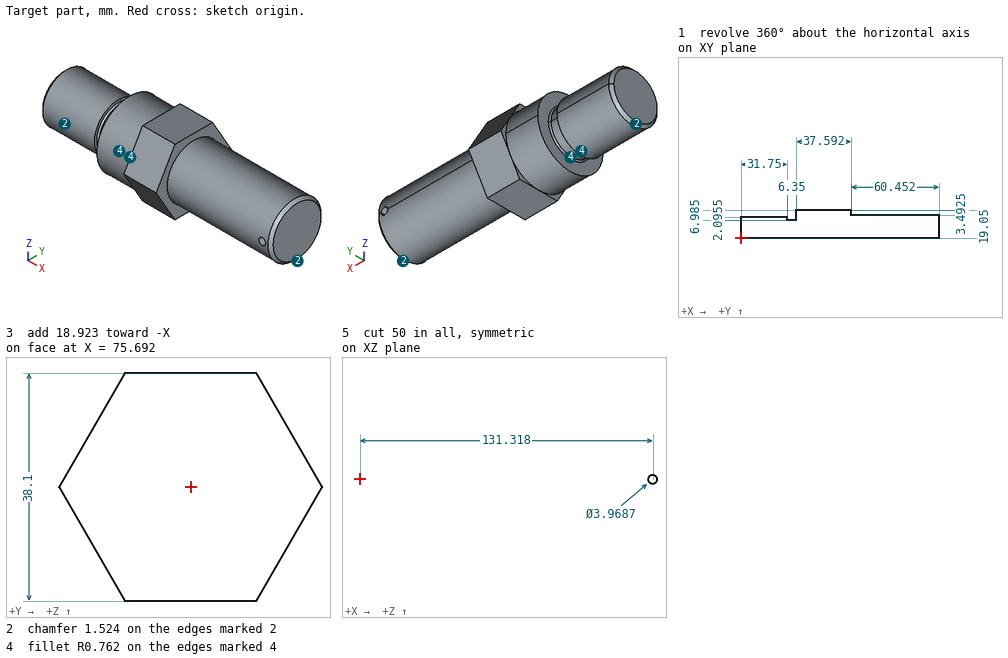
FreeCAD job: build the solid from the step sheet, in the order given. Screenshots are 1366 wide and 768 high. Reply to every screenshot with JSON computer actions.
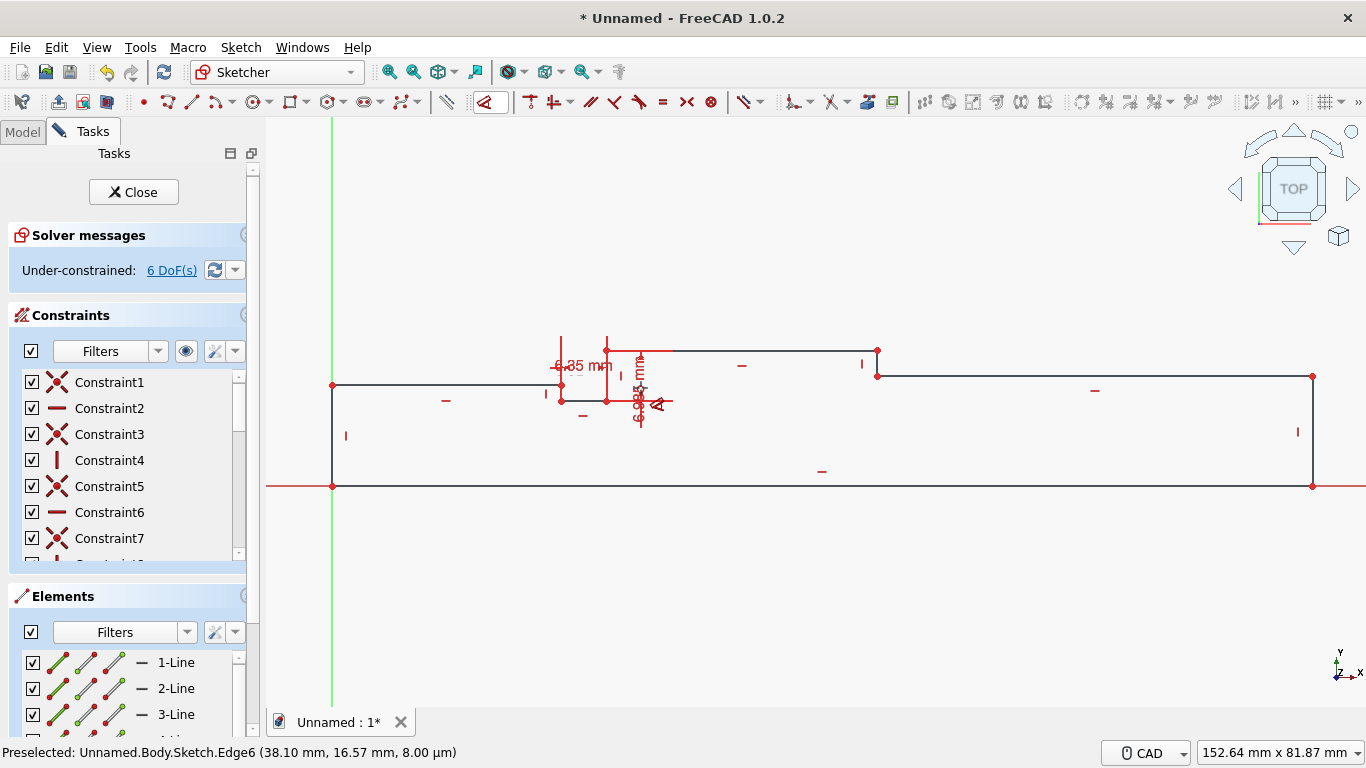
{"action": "left_click", "coordinate": [492, 385]}
{"action": "left_click", "coordinate": [447, 351]}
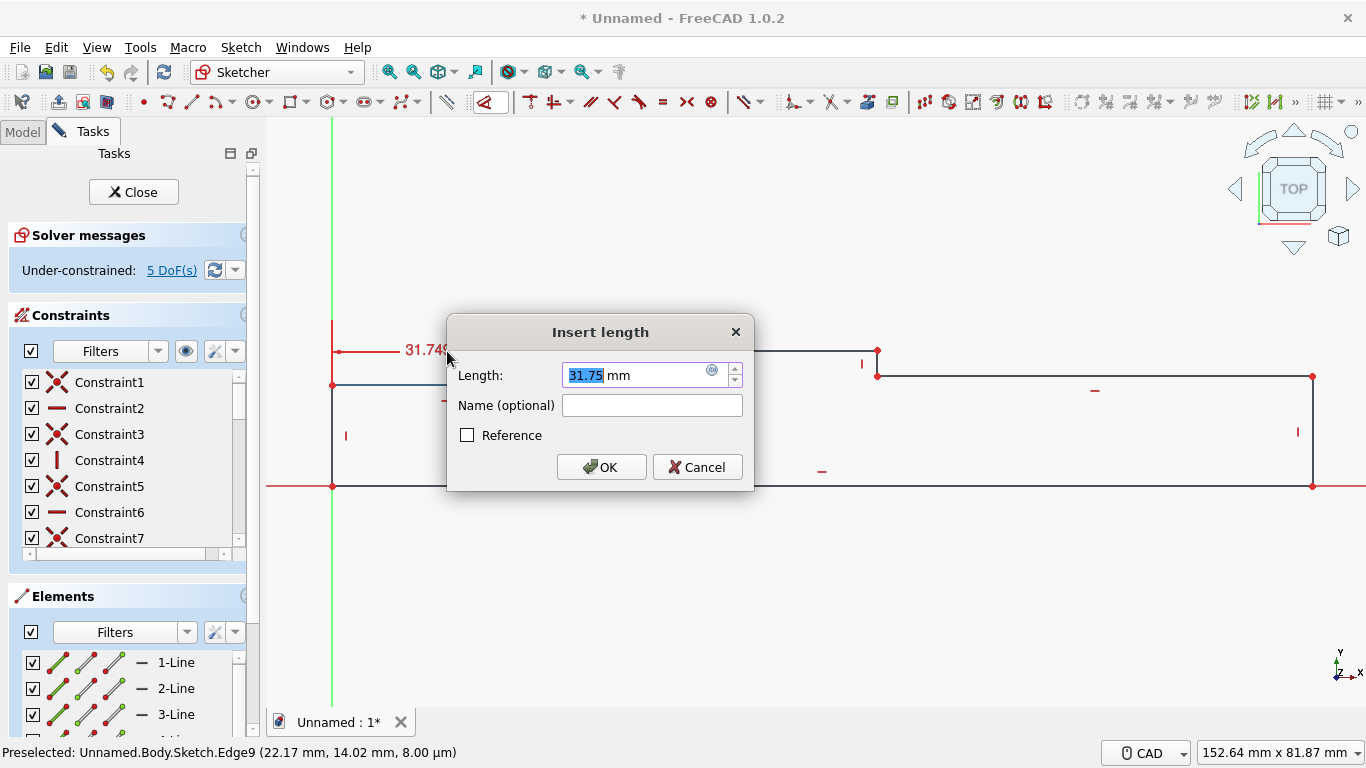
{"action": "type", "text": "31.75"}
{"action": "key", "text": "Return"}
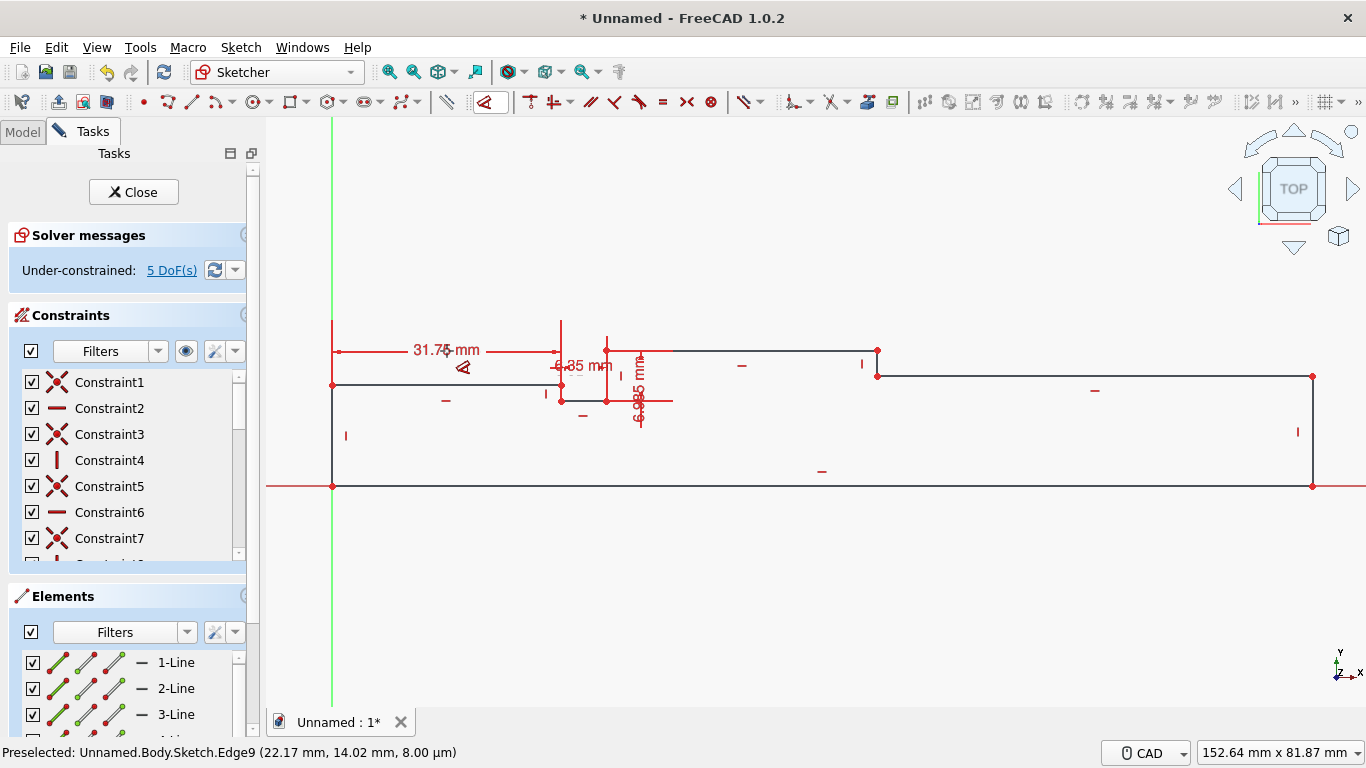
{"action": "left_click", "coordinate": [1182, 376]}
{"action": "left_click", "coordinate": [1039, 342]}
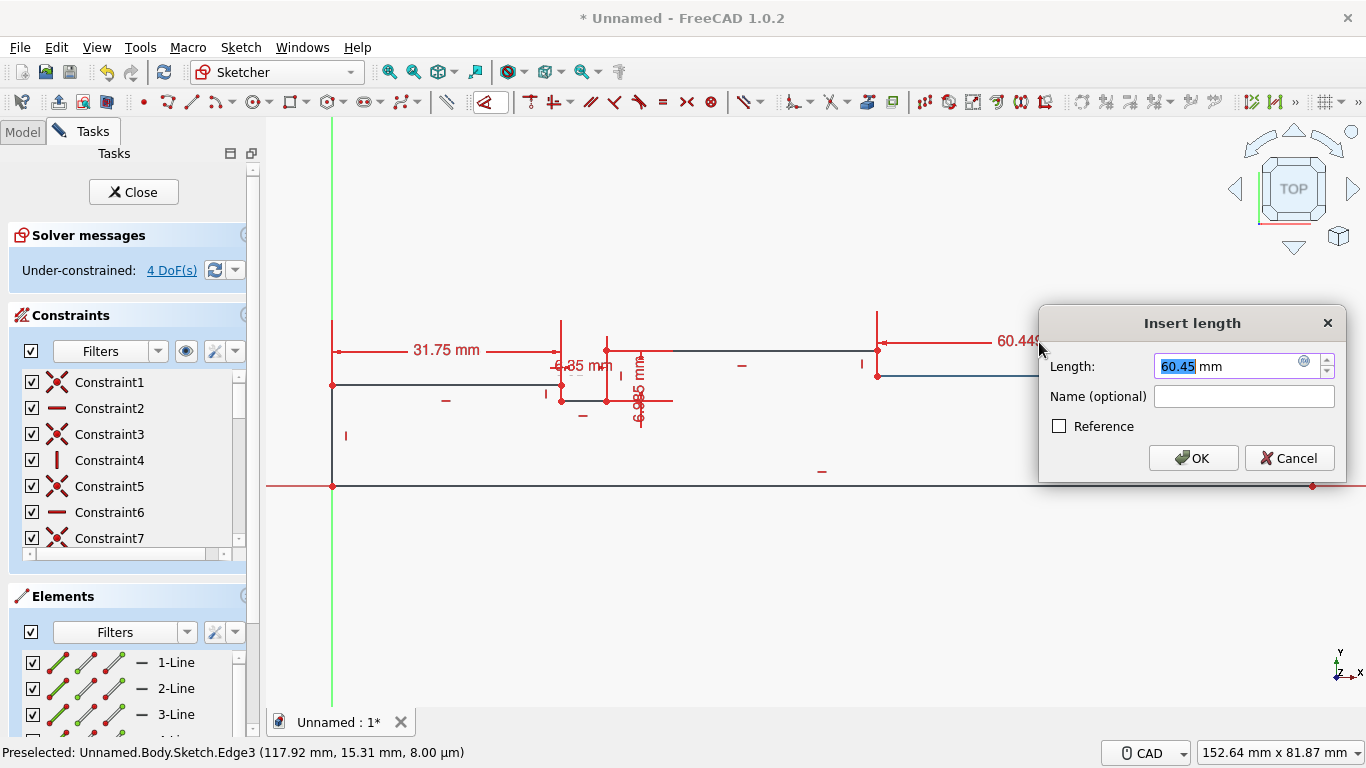
{"action": "type", "text": "60.452"}
{"action": "key", "text": "Return"}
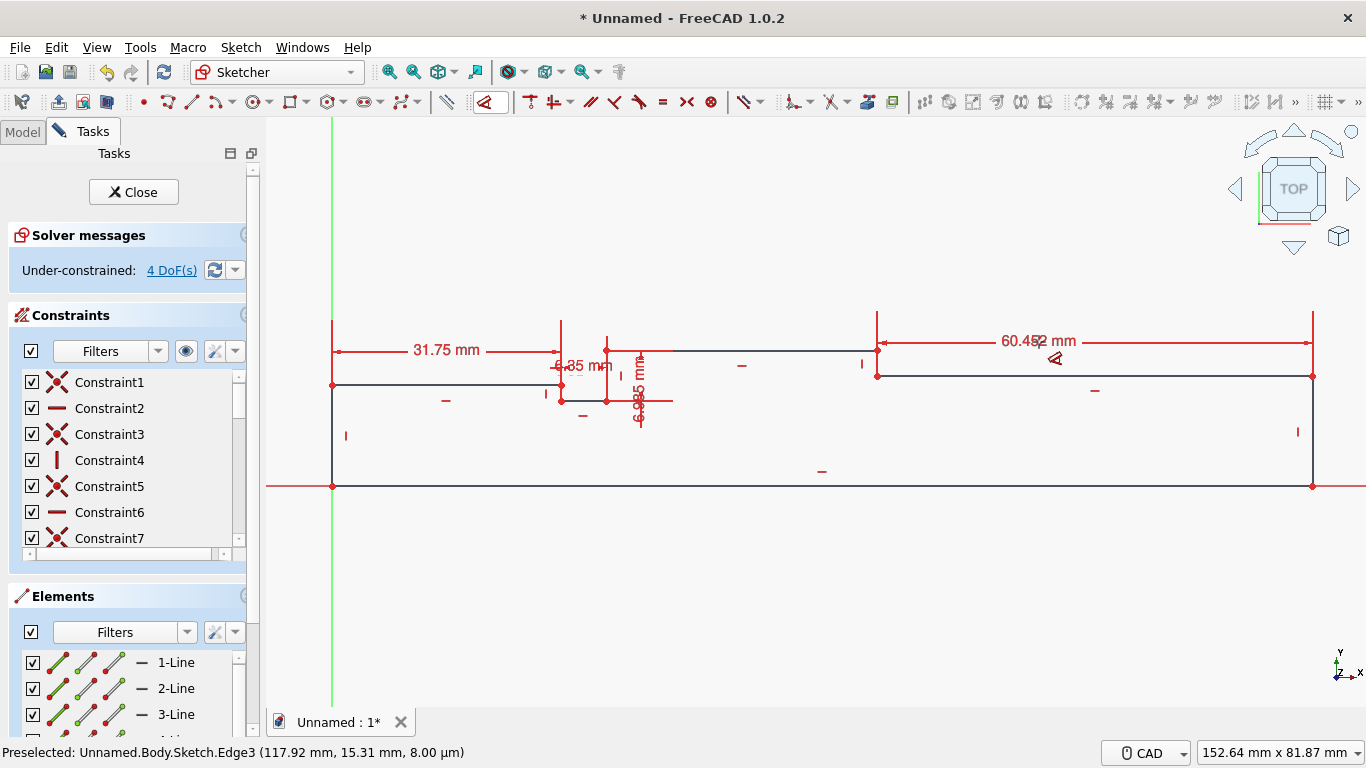
{"action": "scroll", "coordinate": [877, 366], "scroll_direction": "up", "scroll_amount": 3}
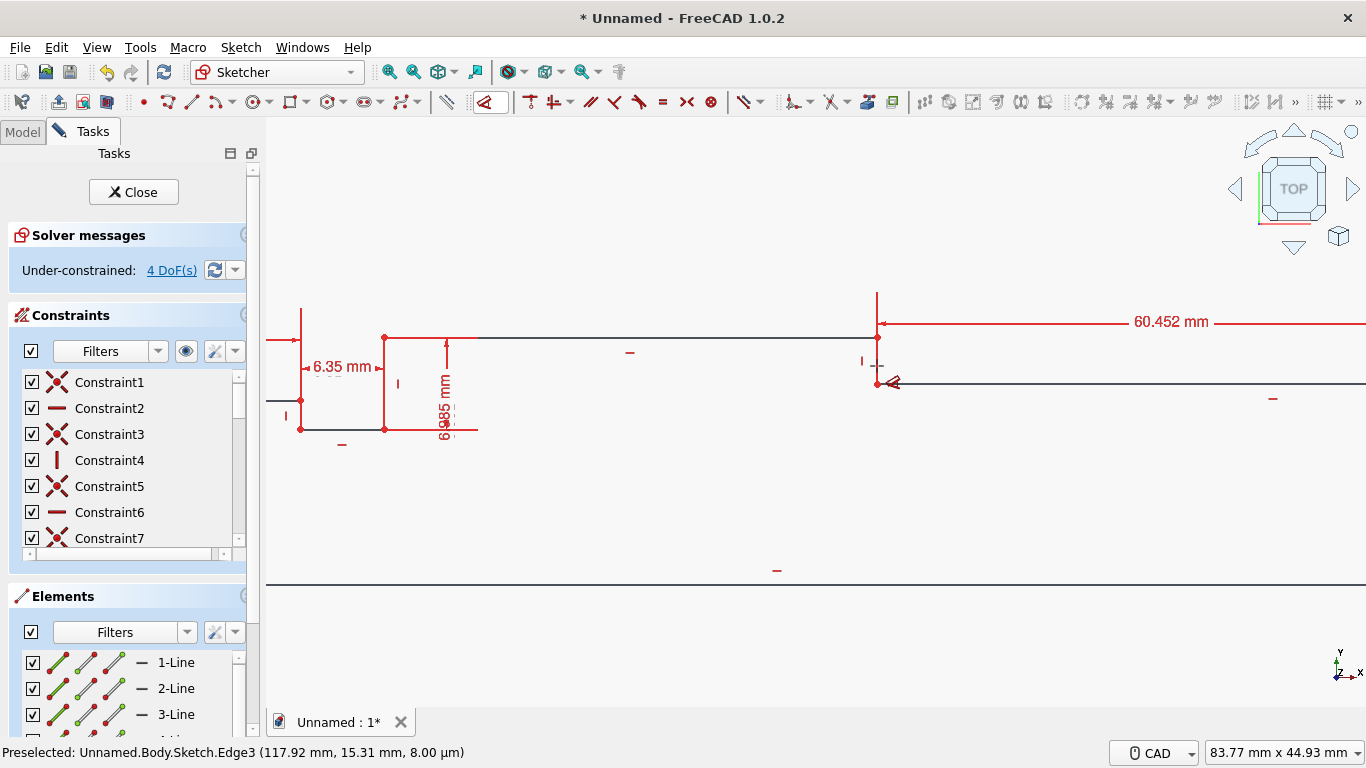
{"action": "left_click", "coordinate": [877, 366]}
{"action": "left_click", "coordinate": [911, 361]}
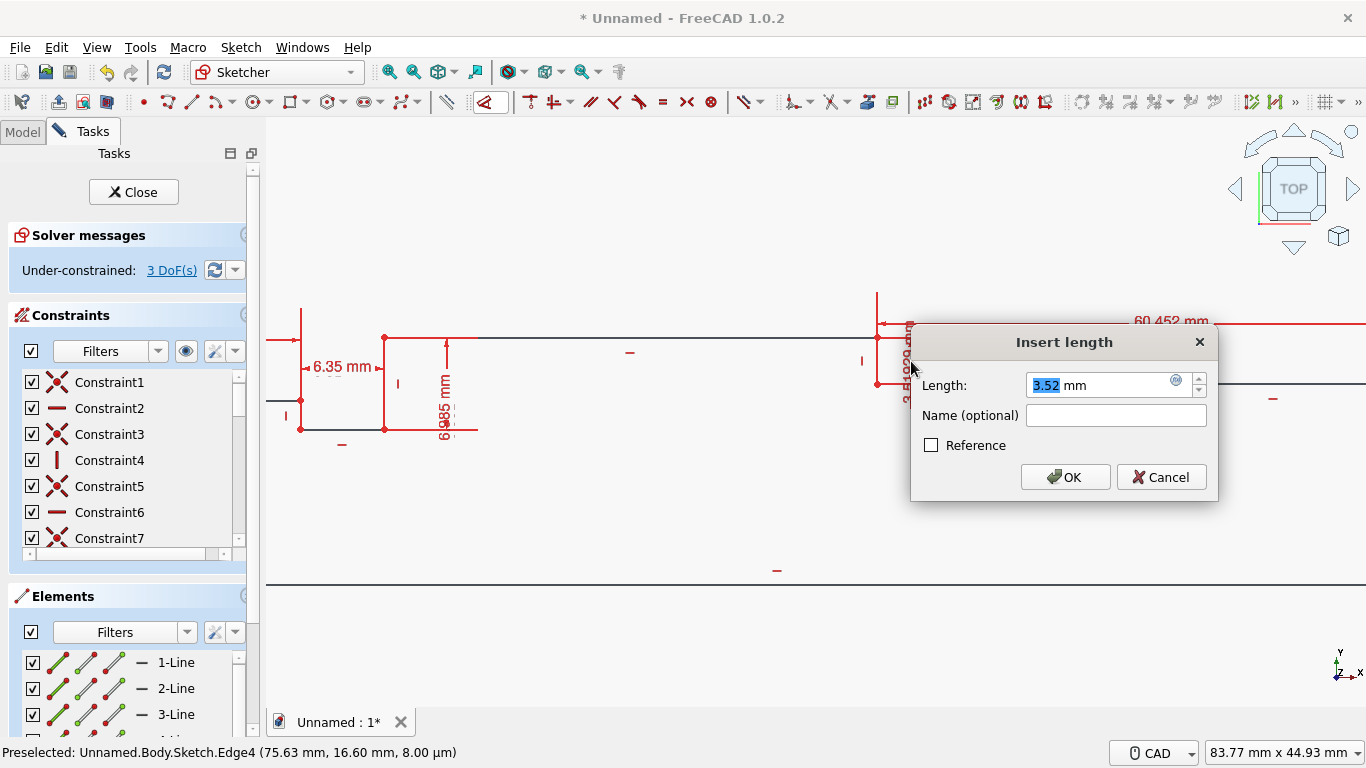
{"action": "type", "text": "3.4925"}
{"action": "key", "text": "Return"}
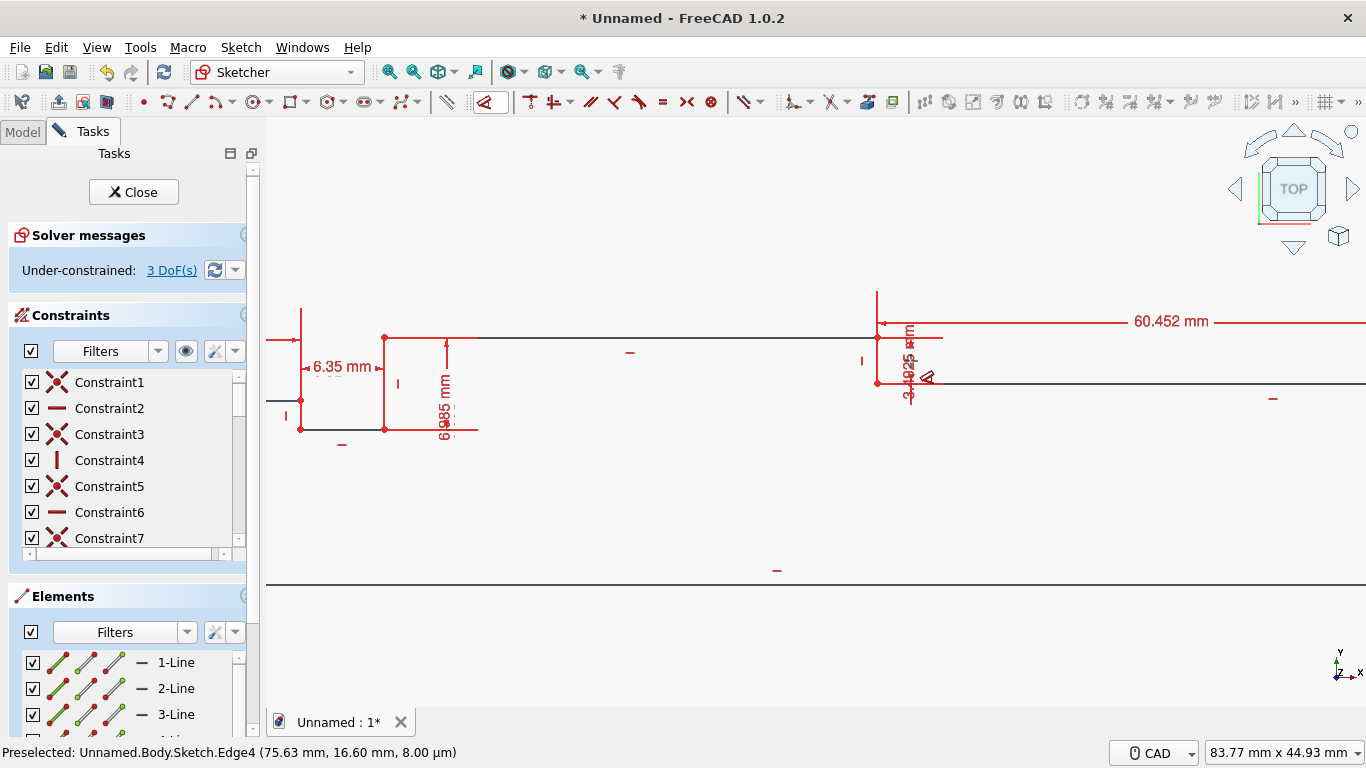
{"action": "left_click", "coordinate": [729, 338]}
{"action": "left_click", "coordinate": [631, 304]}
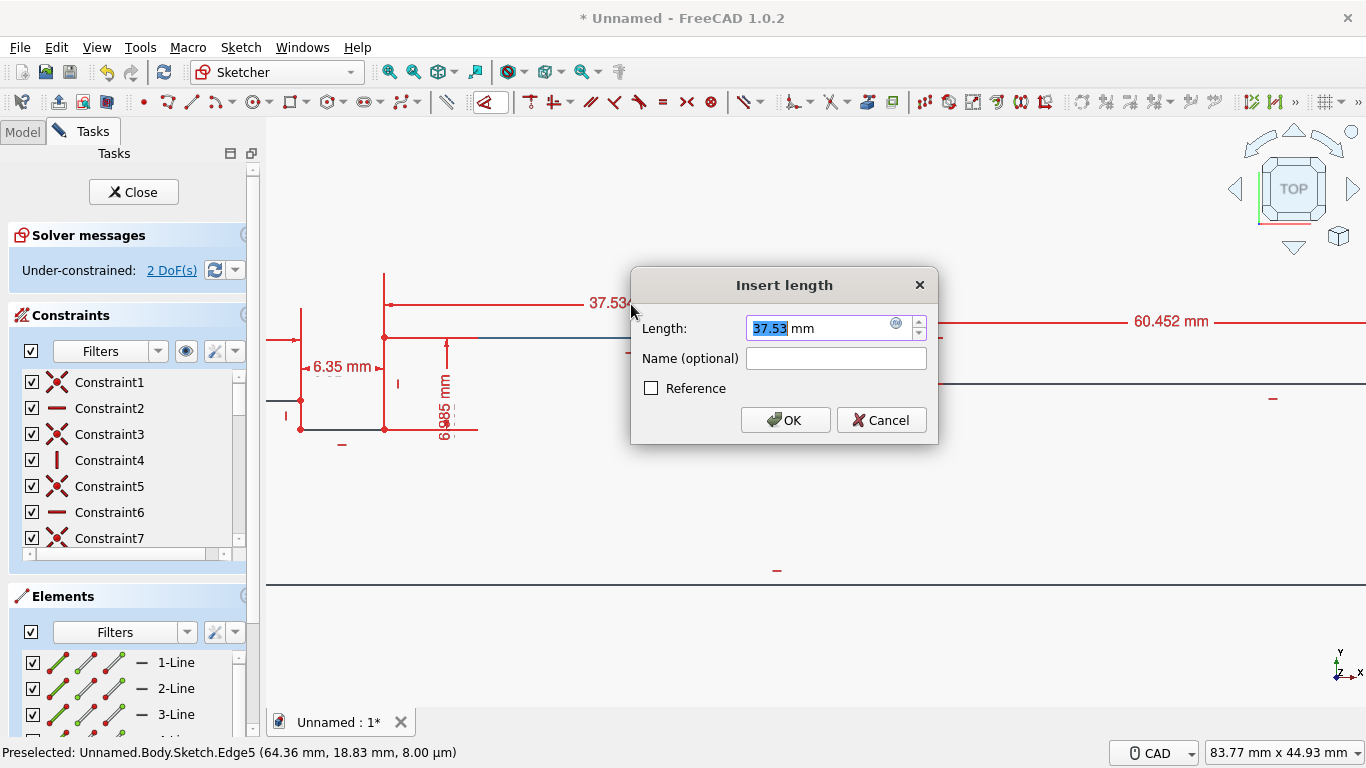
{"action": "type", "text": "37.592"}
{"action": "key", "text": "Return"}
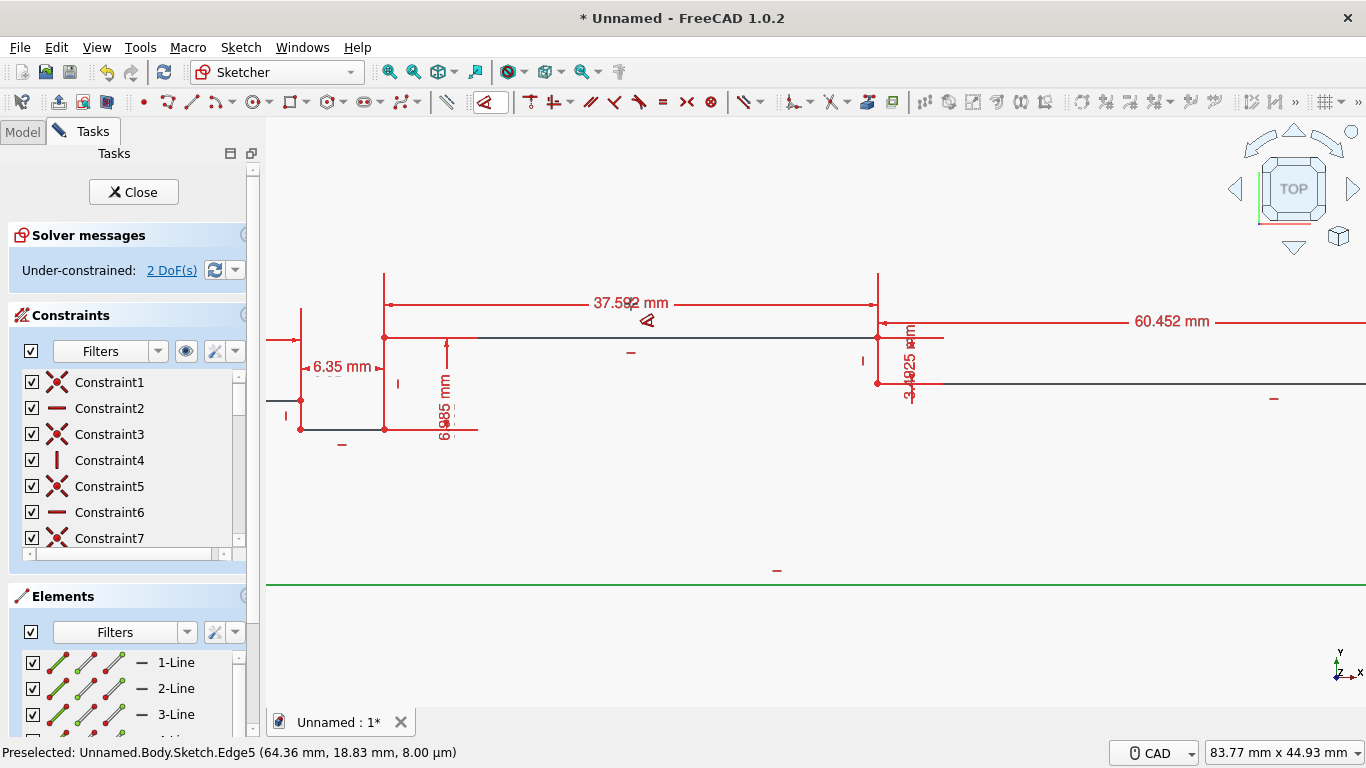
{"action": "scroll", "coordinate": [301, 418], "scroll_direction": "up", "scroll_amount": 2}